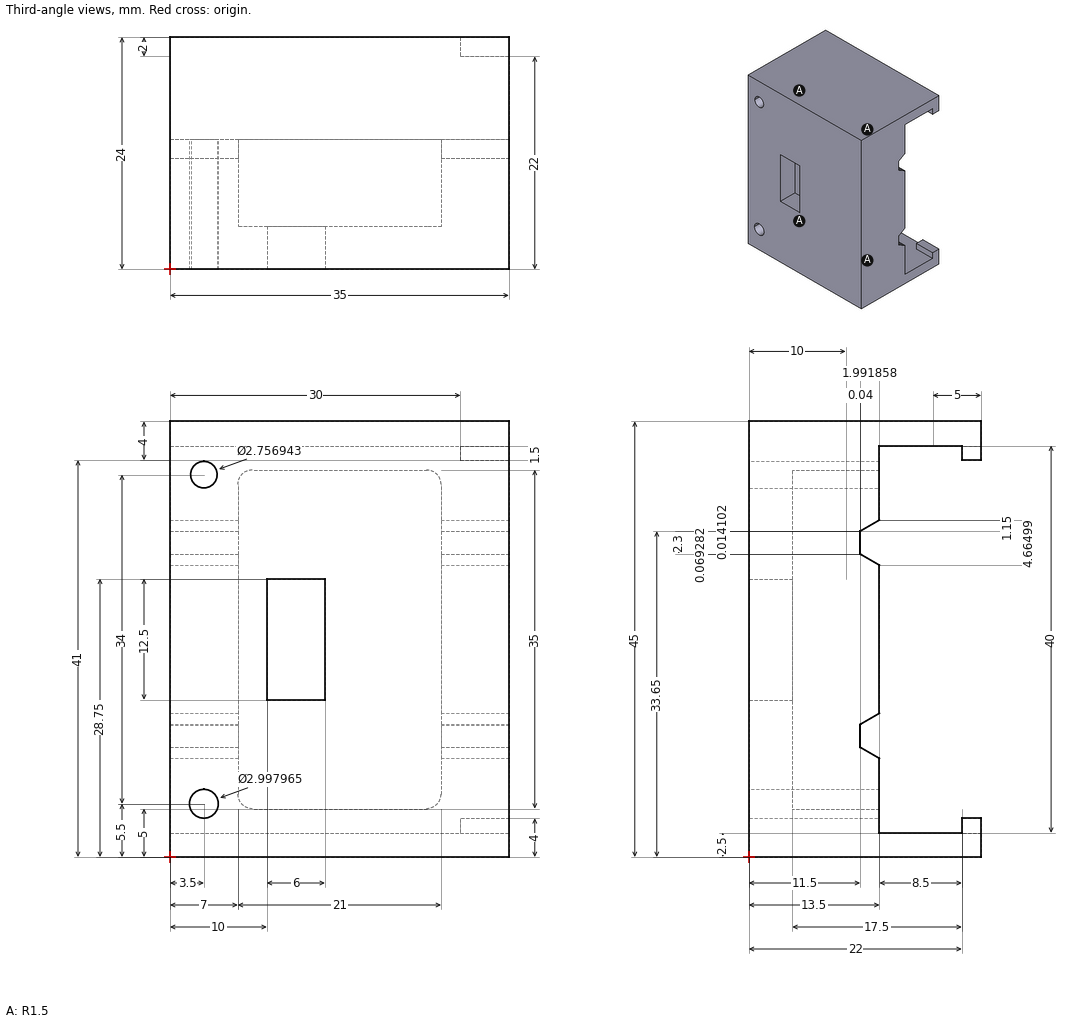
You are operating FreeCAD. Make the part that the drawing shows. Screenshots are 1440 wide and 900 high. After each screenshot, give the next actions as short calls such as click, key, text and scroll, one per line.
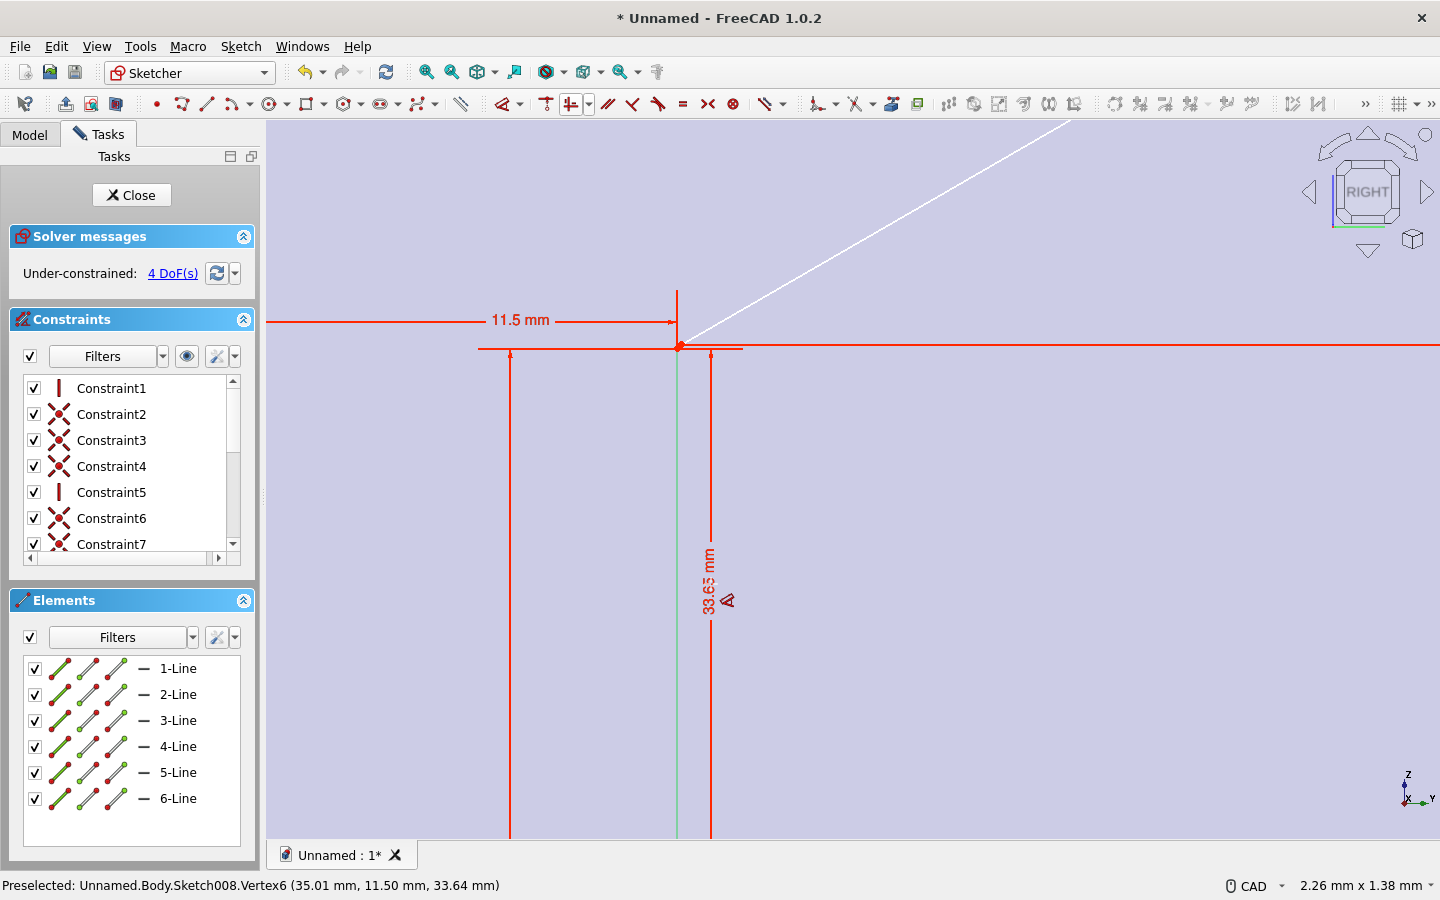
scroll(680, 359, down, 8)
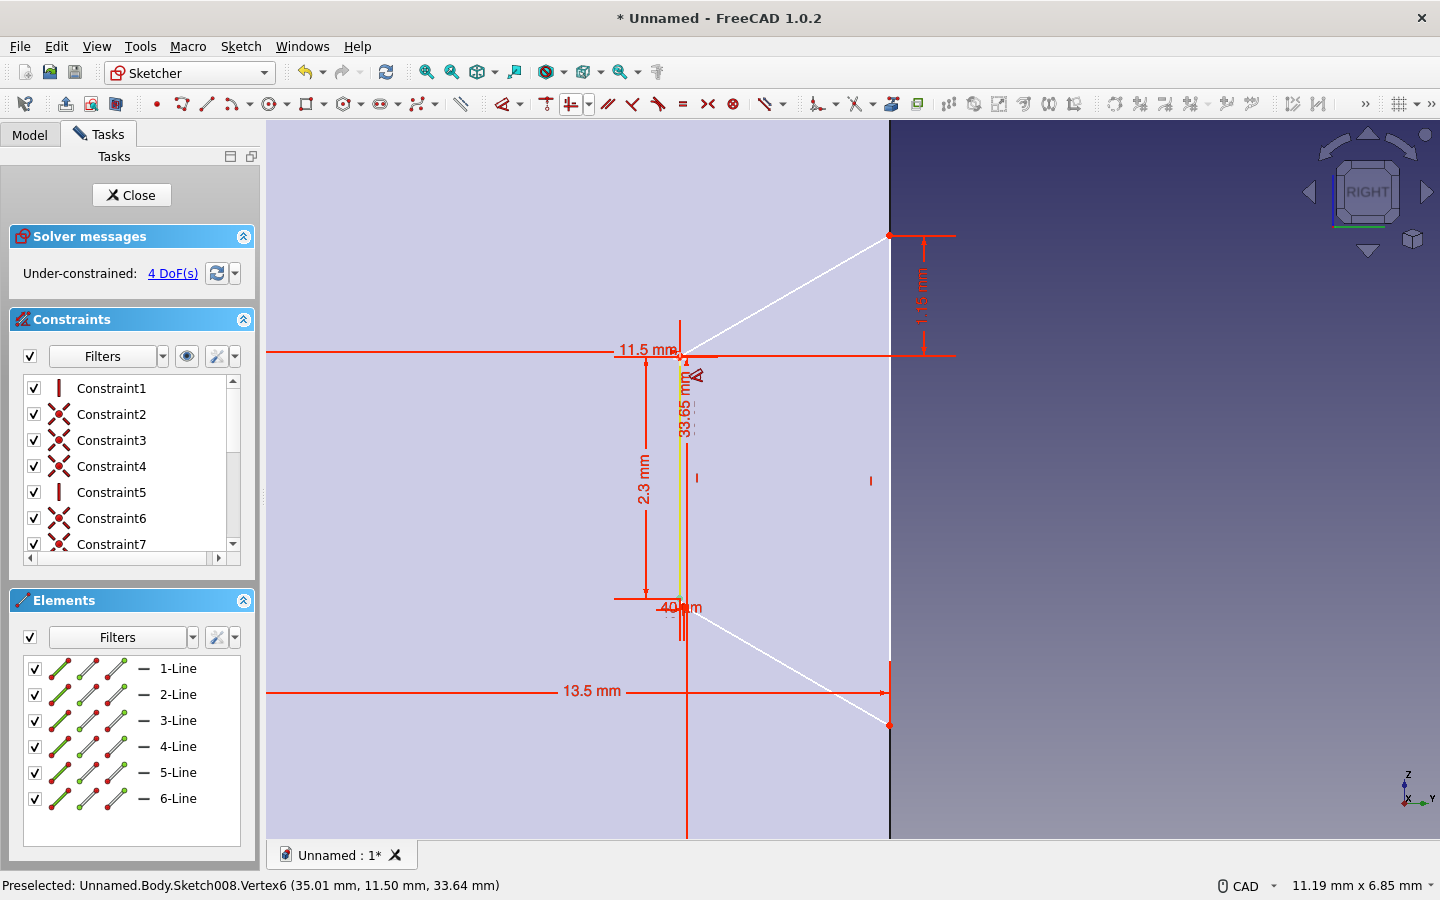
click(890, 579)
click(924, 481)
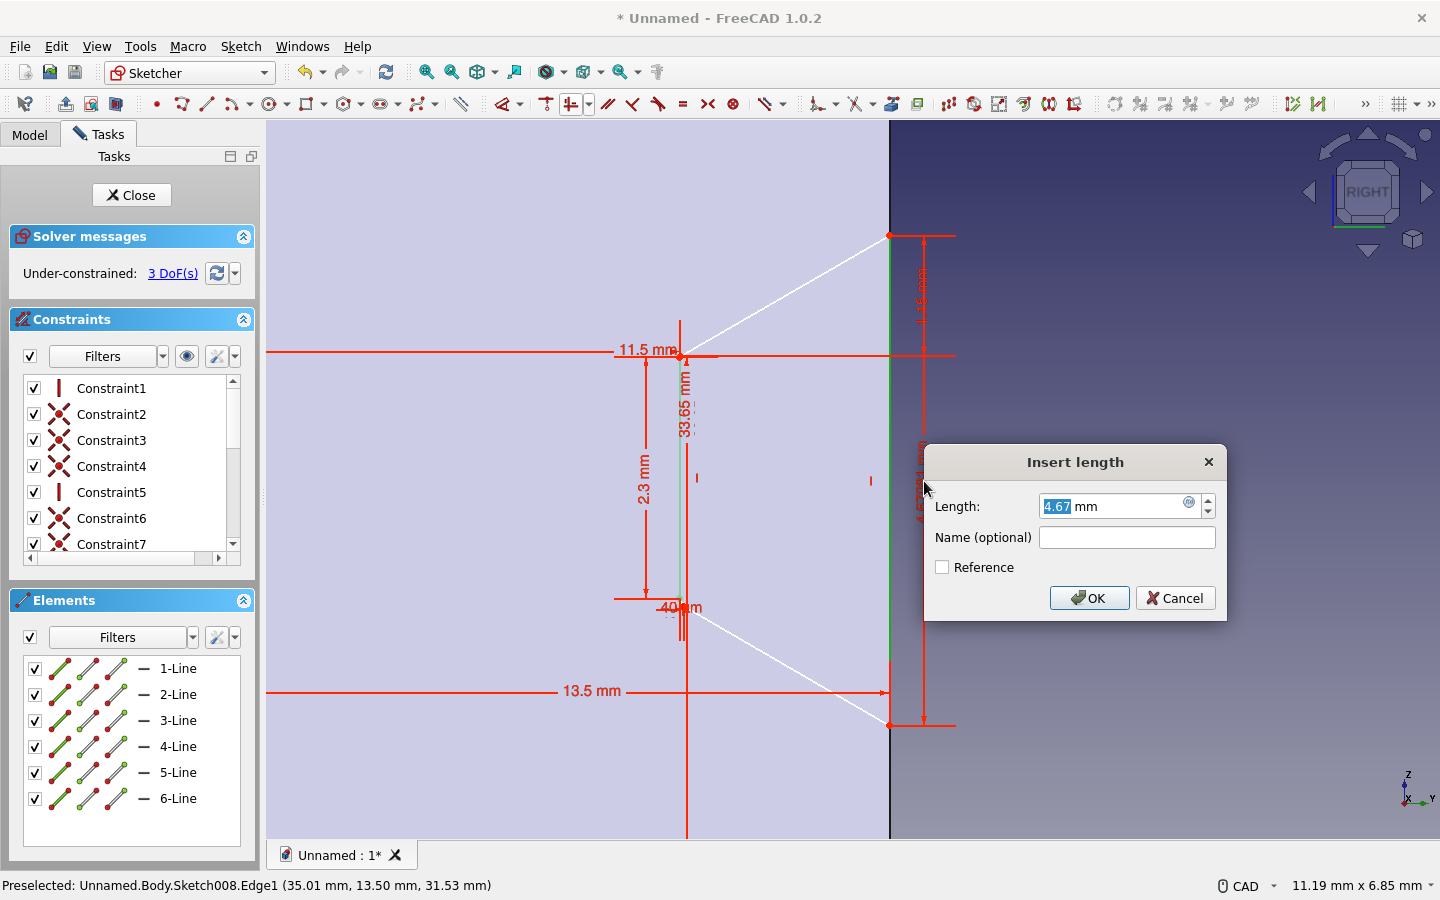
text(4.66499)
key(Return)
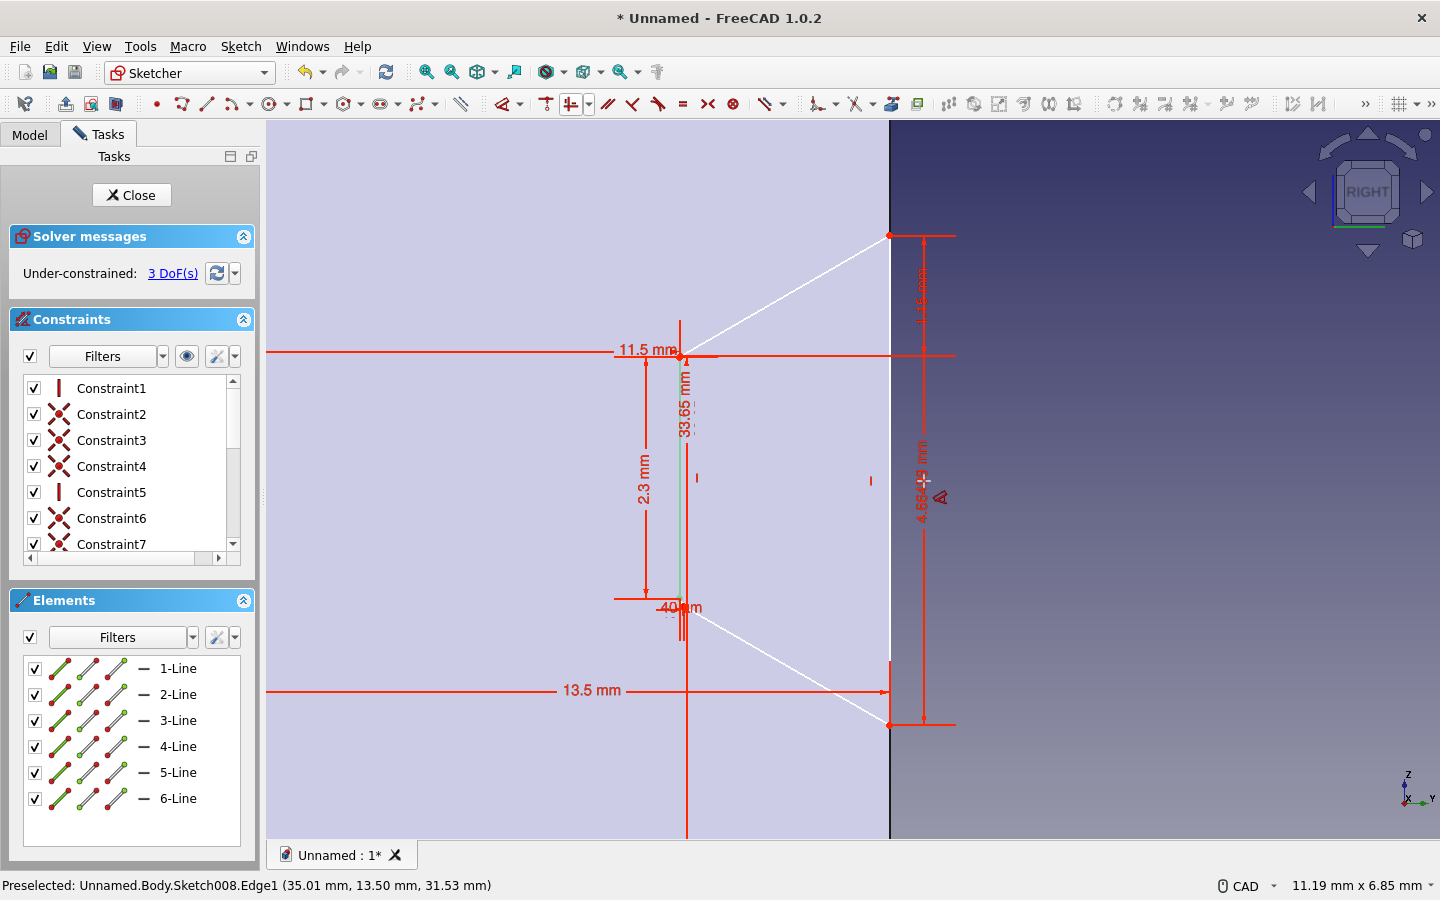
click(827, 272)
click(785, 202)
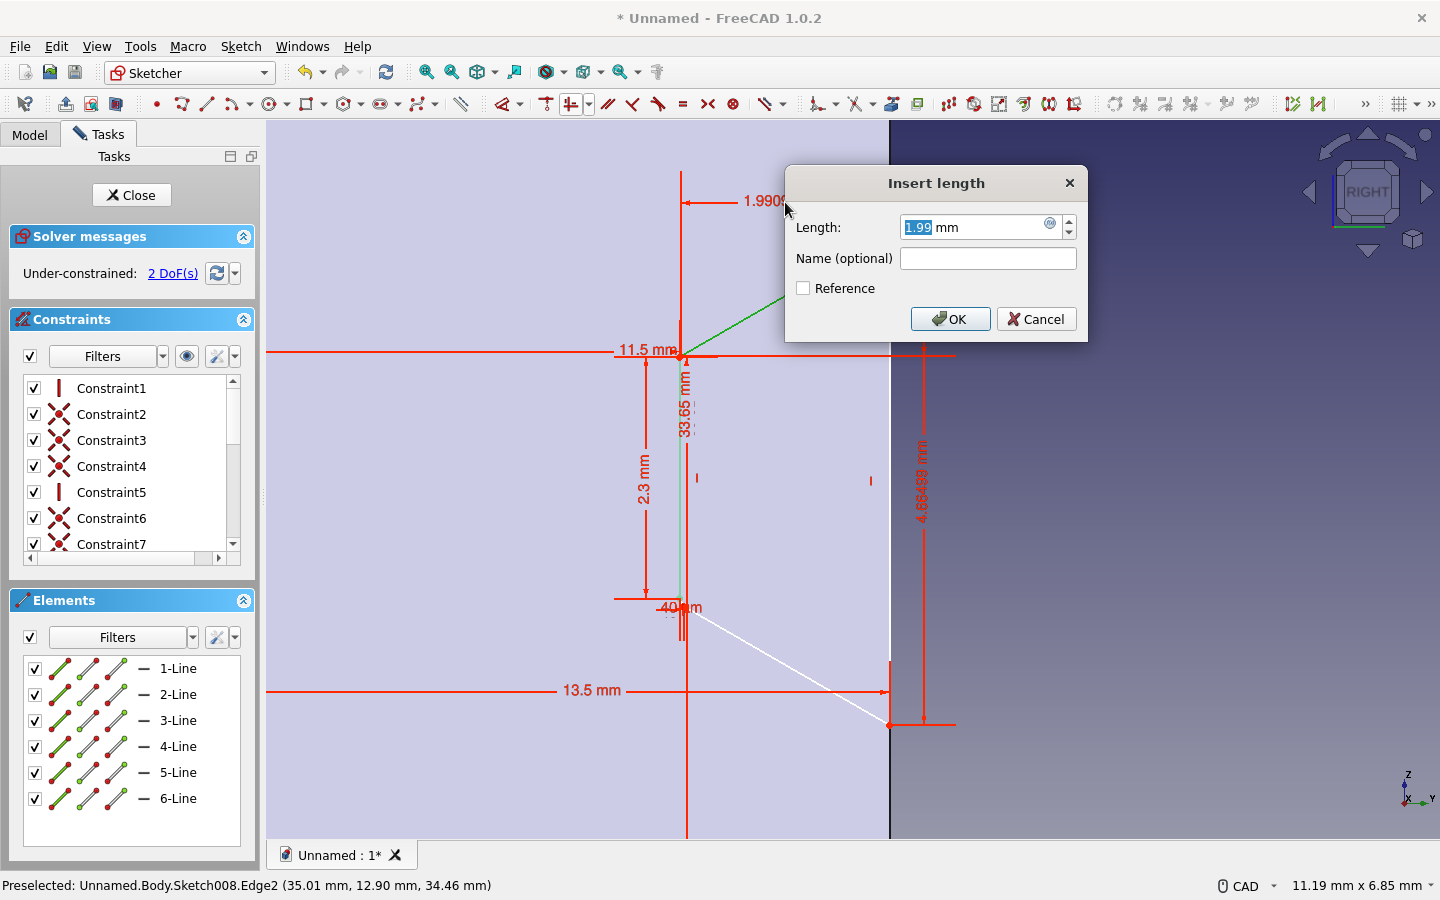
text(1.991858)
key(Return)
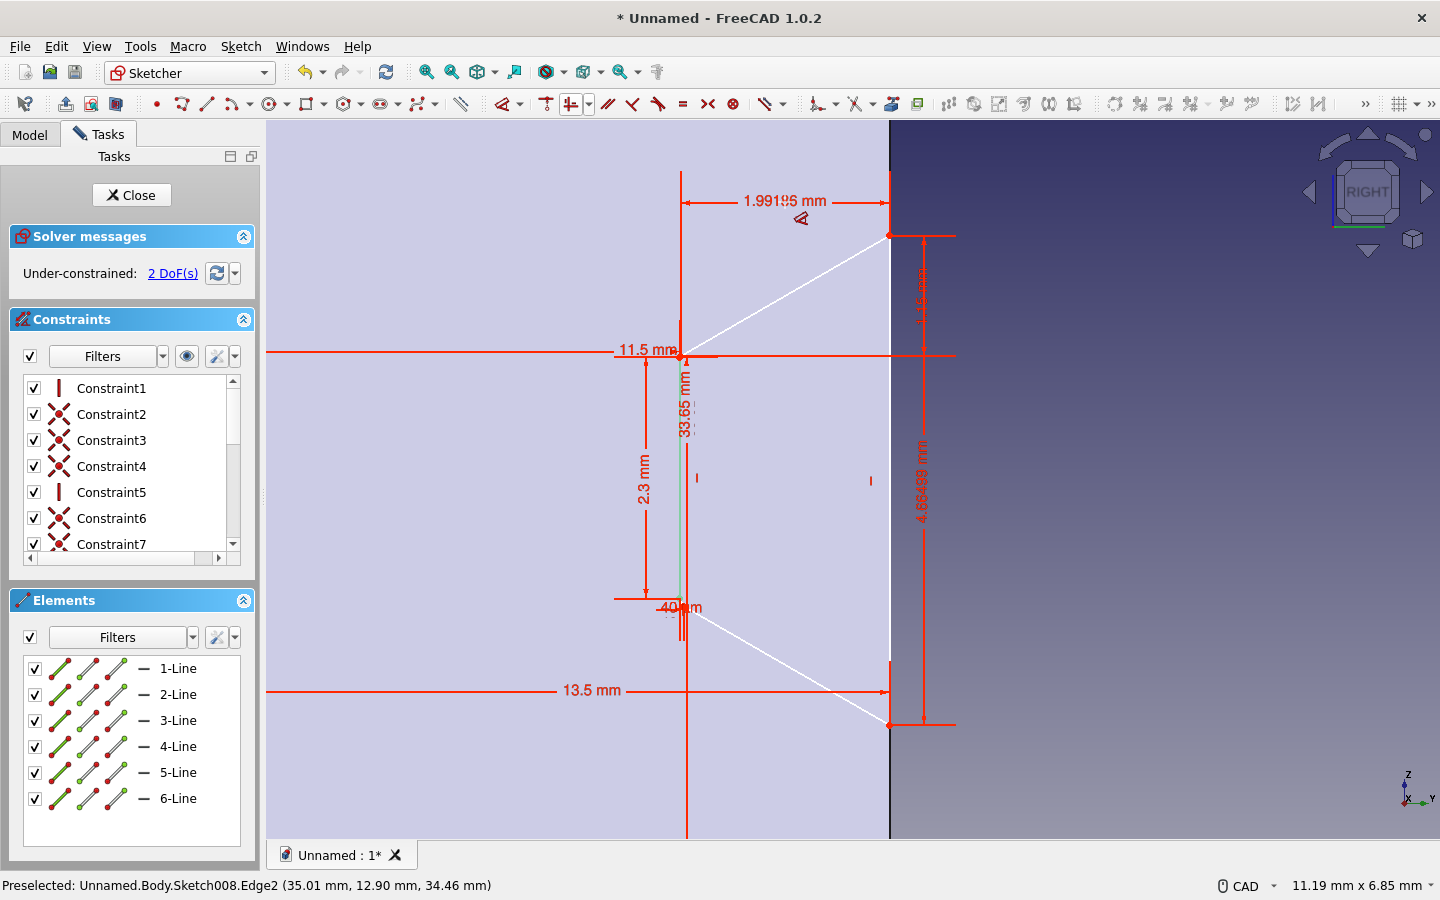
scroll(680, 357, up, 17)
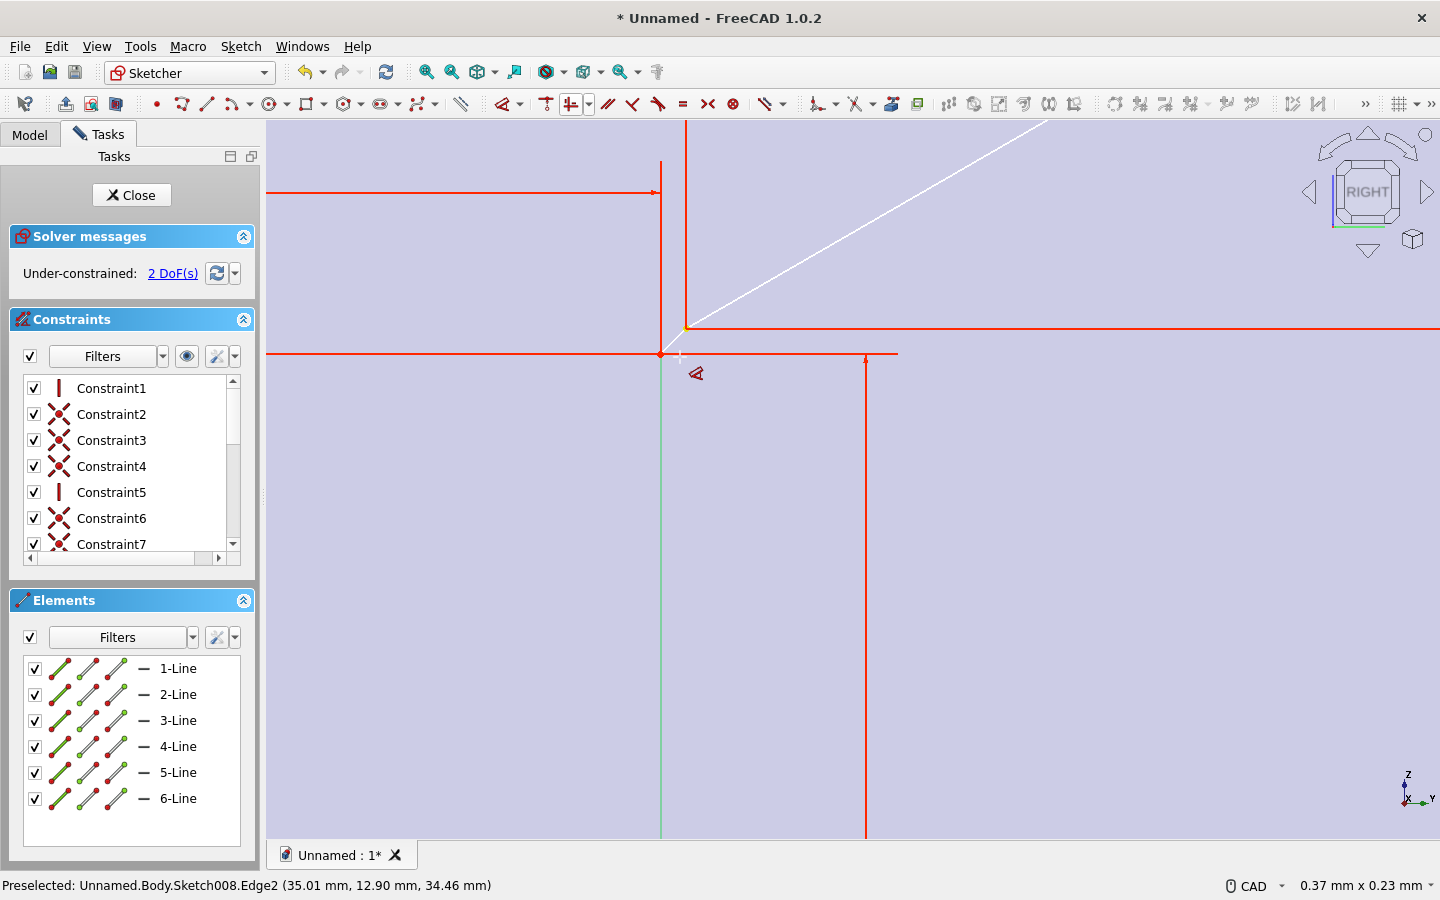
click(673, 341)
click(627, 341)